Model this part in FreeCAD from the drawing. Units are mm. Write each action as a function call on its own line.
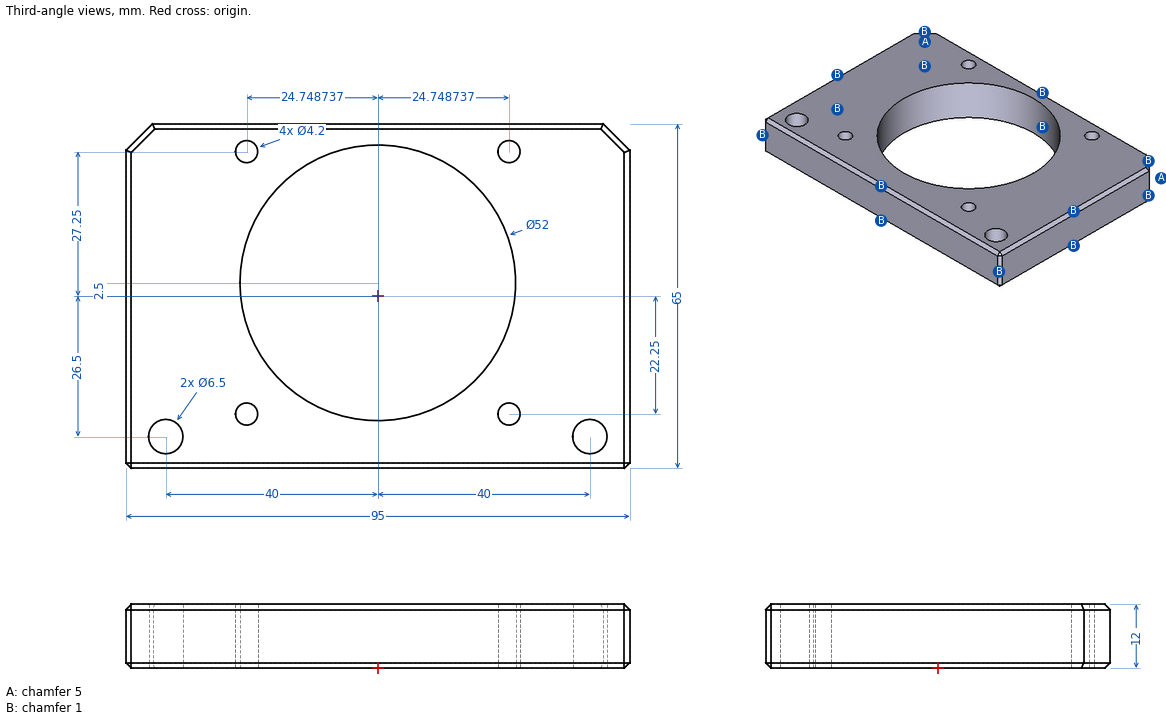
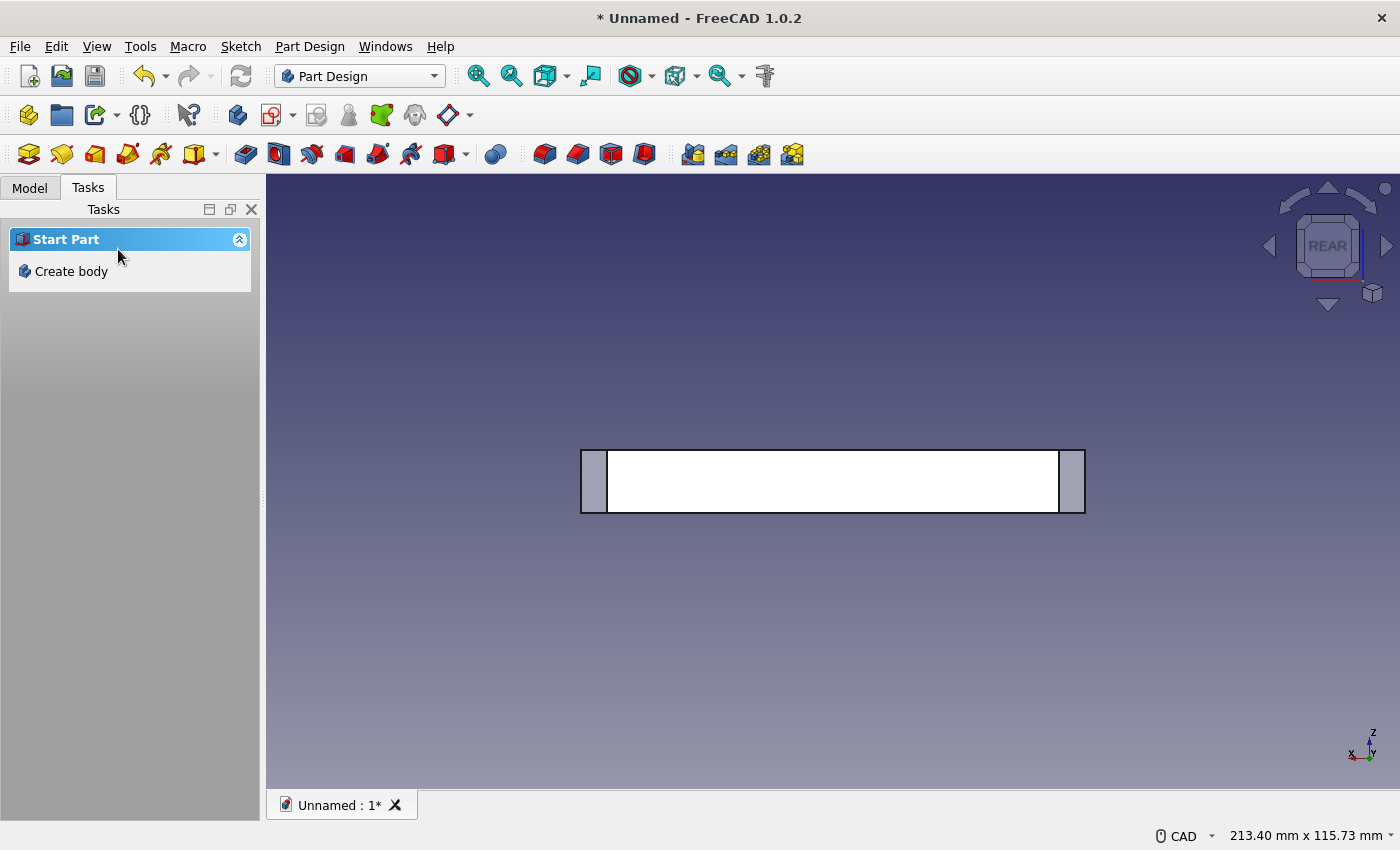
key(0)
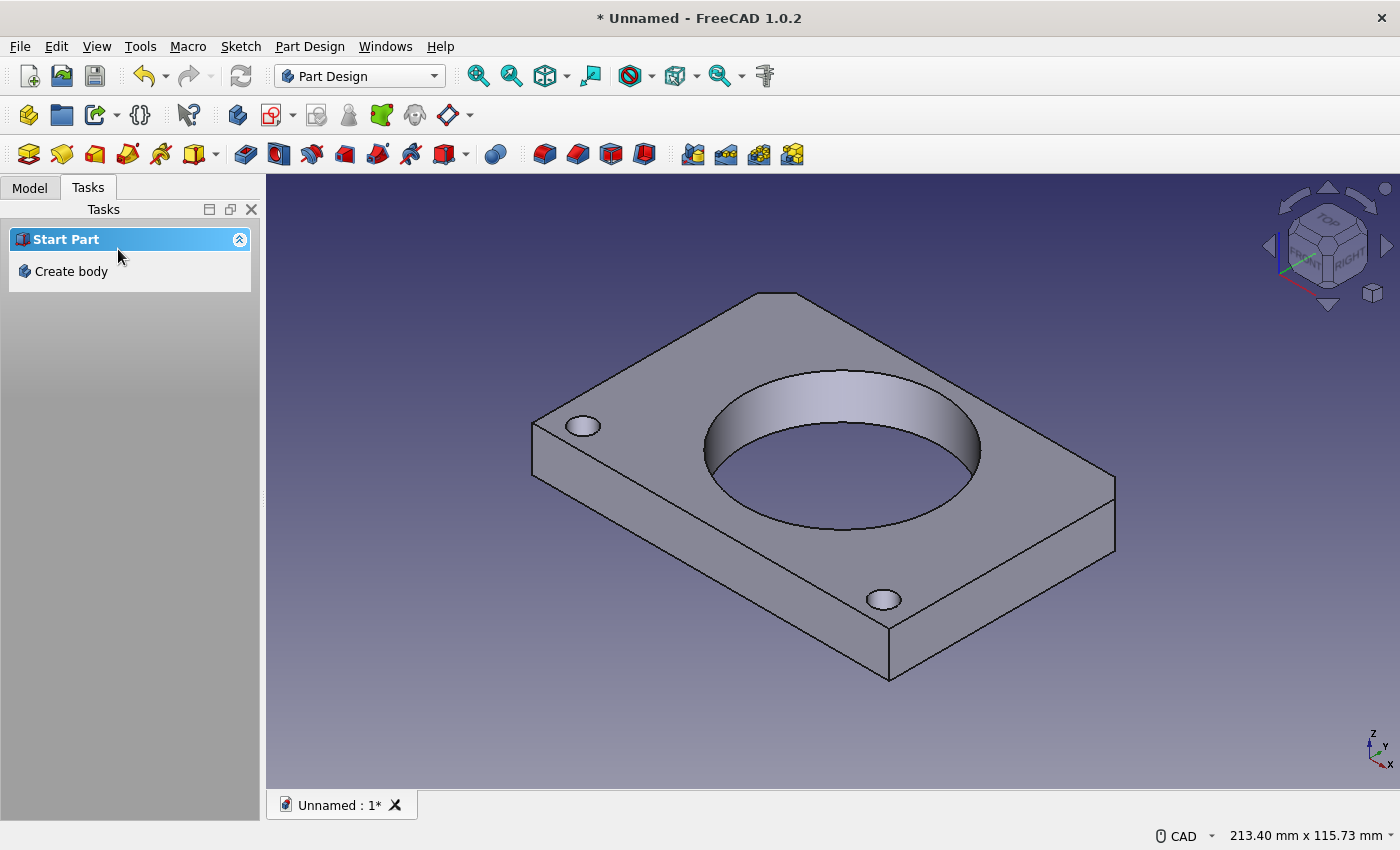
click(661, 436)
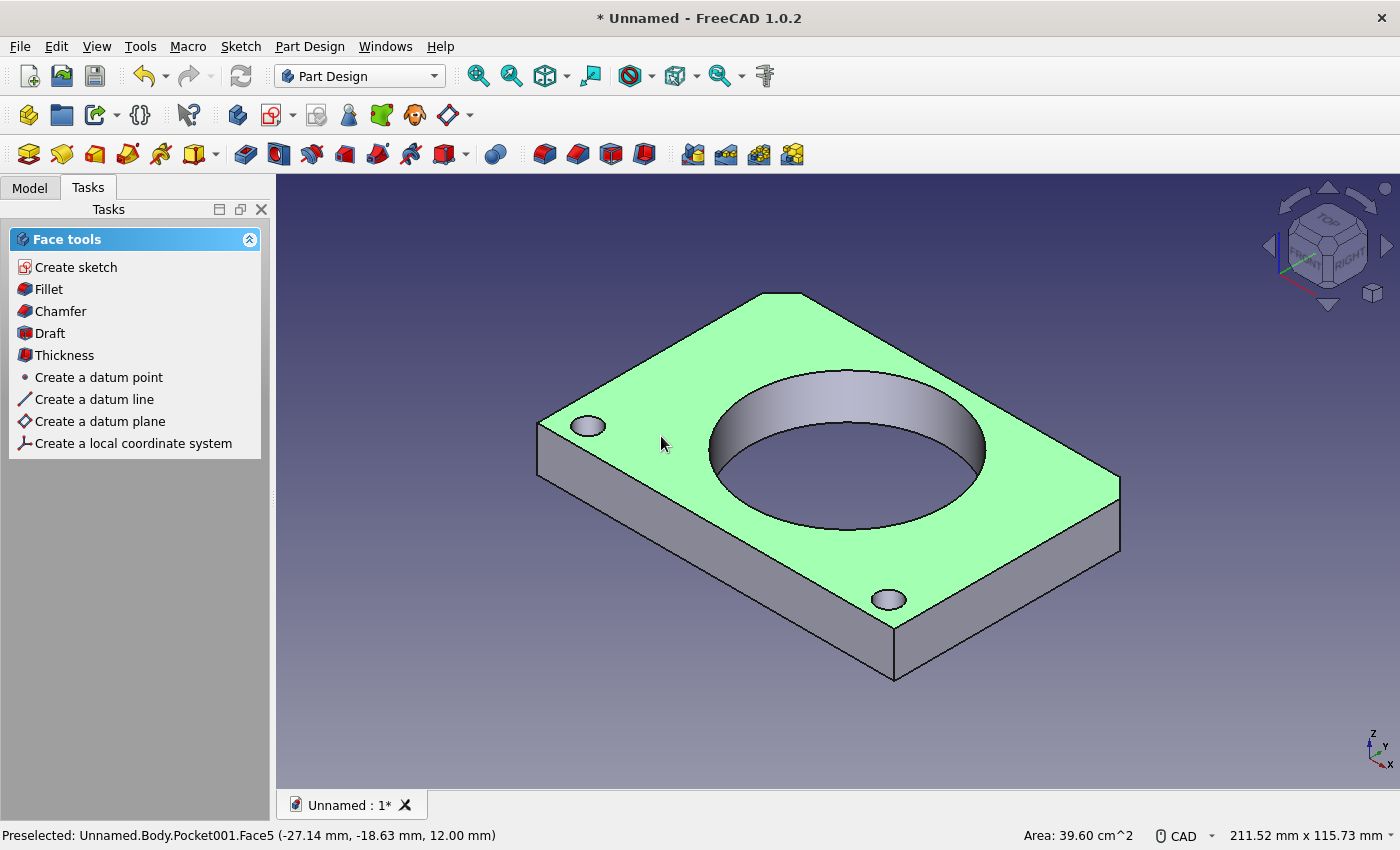
click(270, 116)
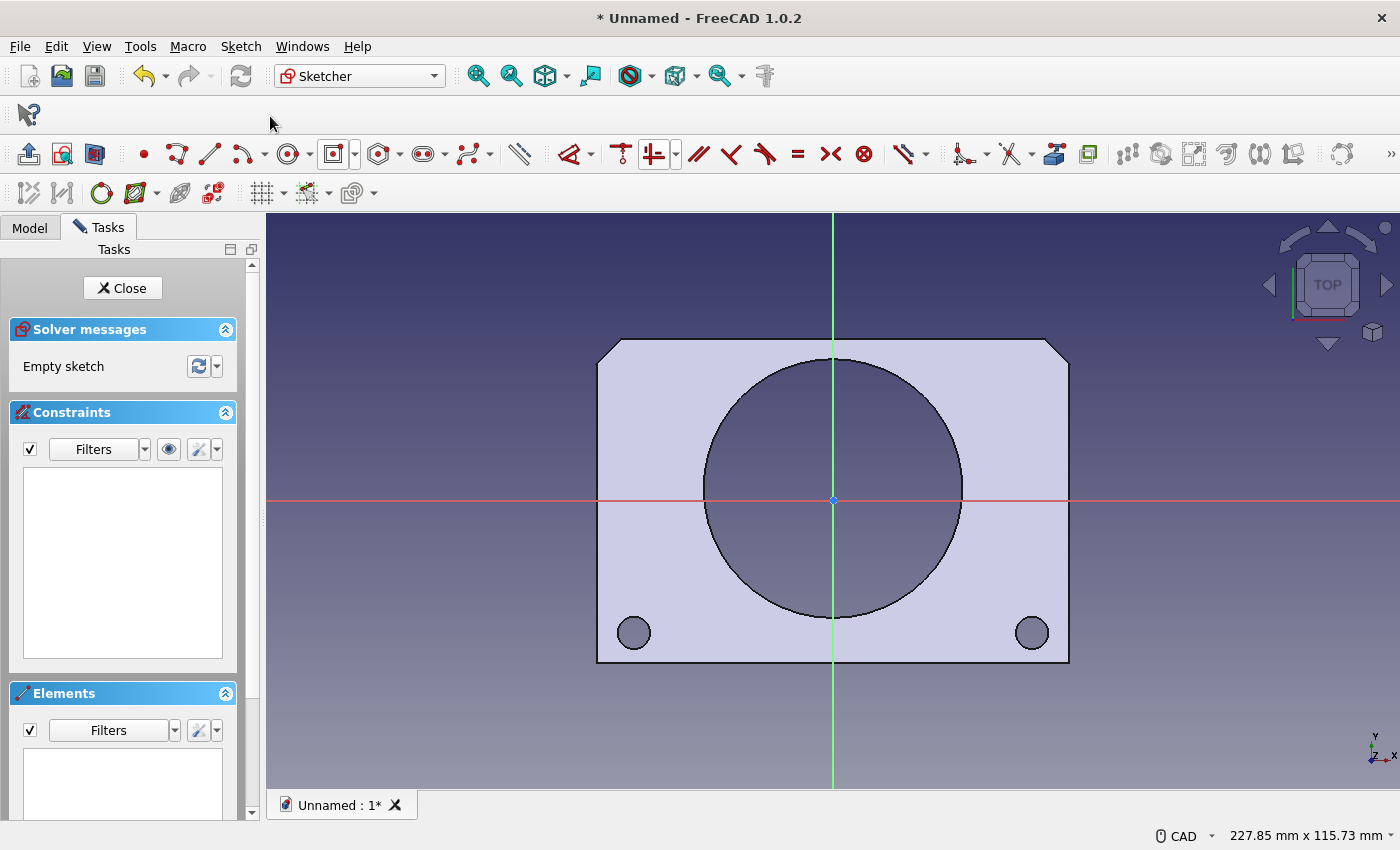
scroll(972, 463, up, 2)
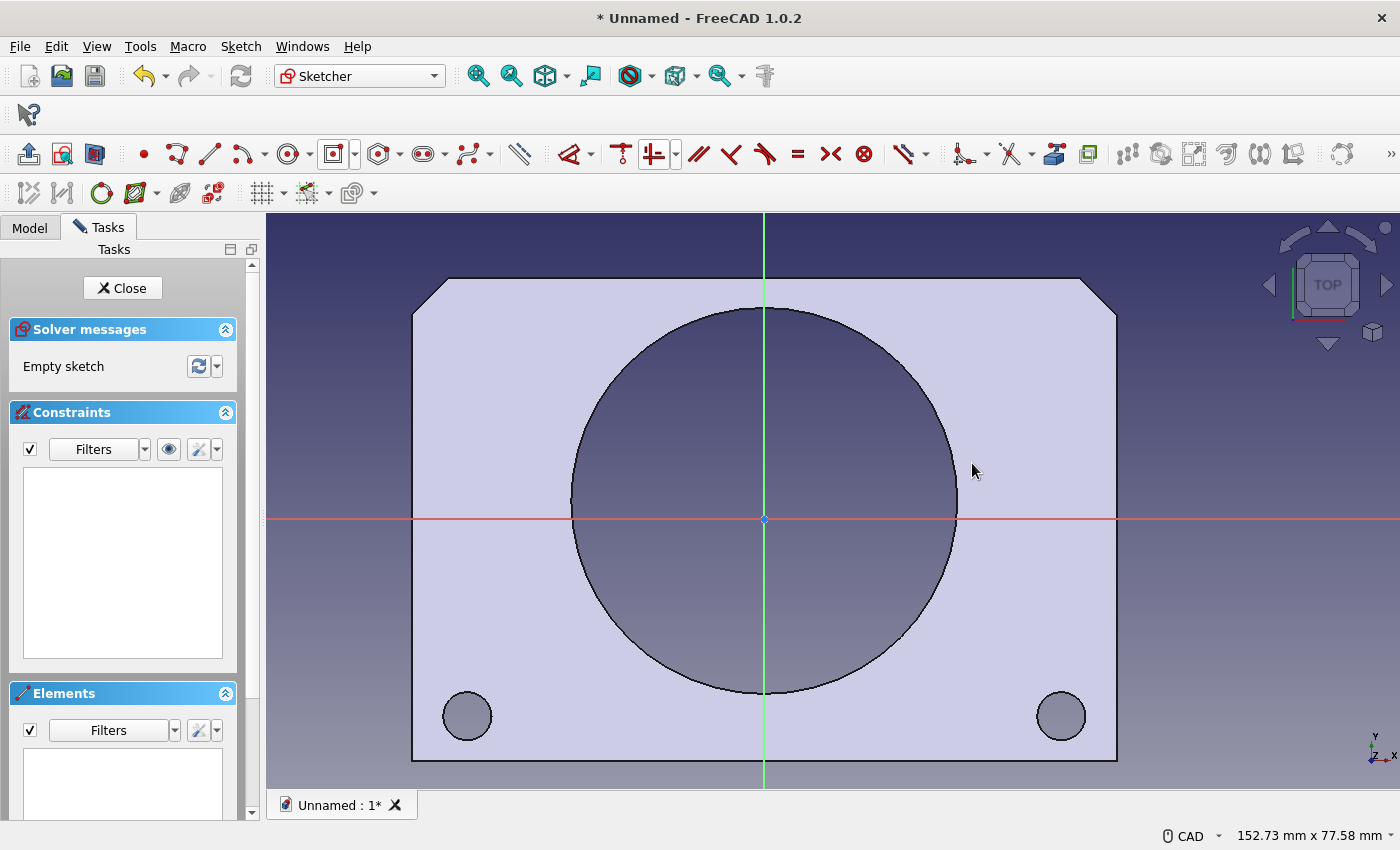
click(288, 154)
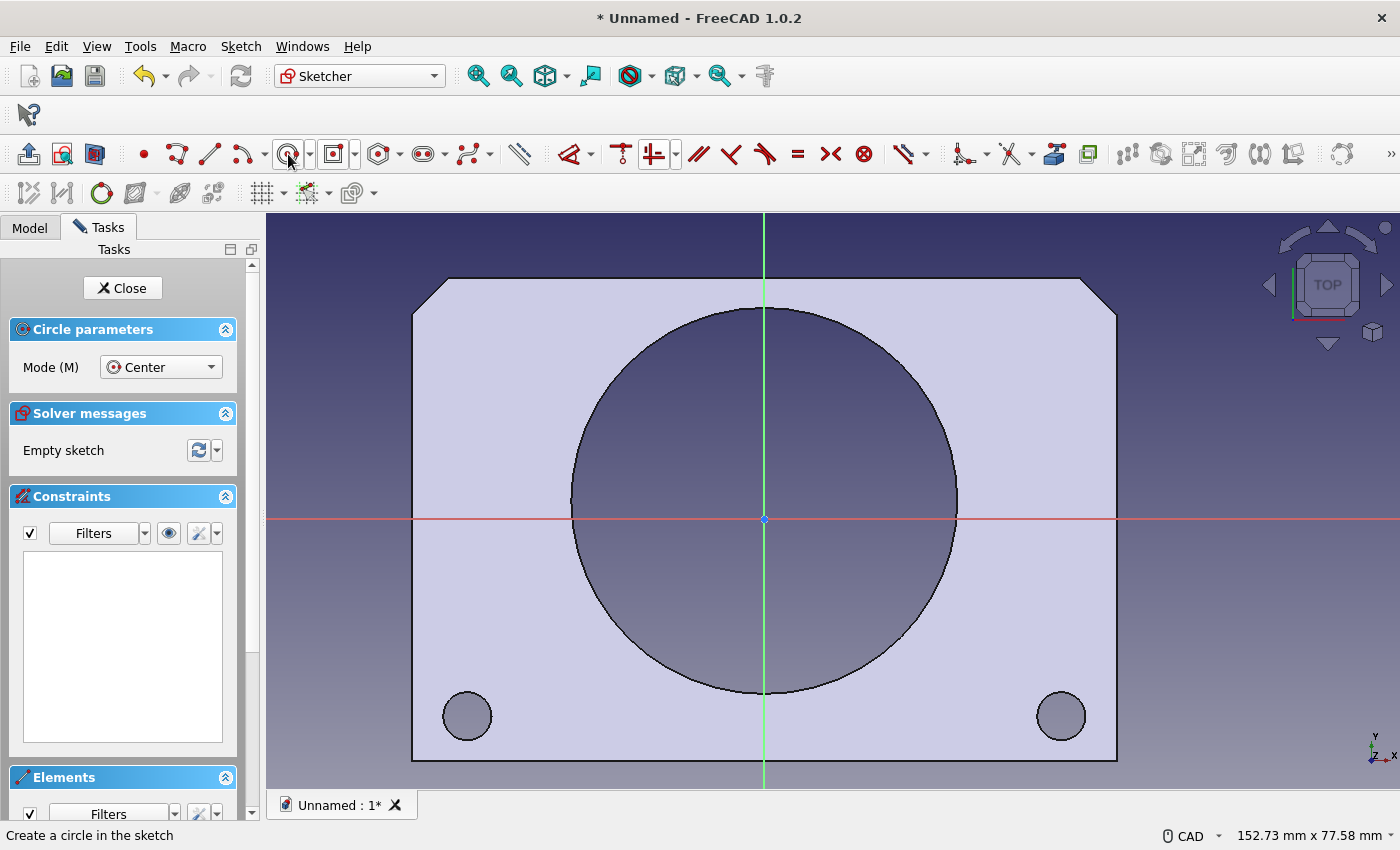
scroll(581, 317, up, 2)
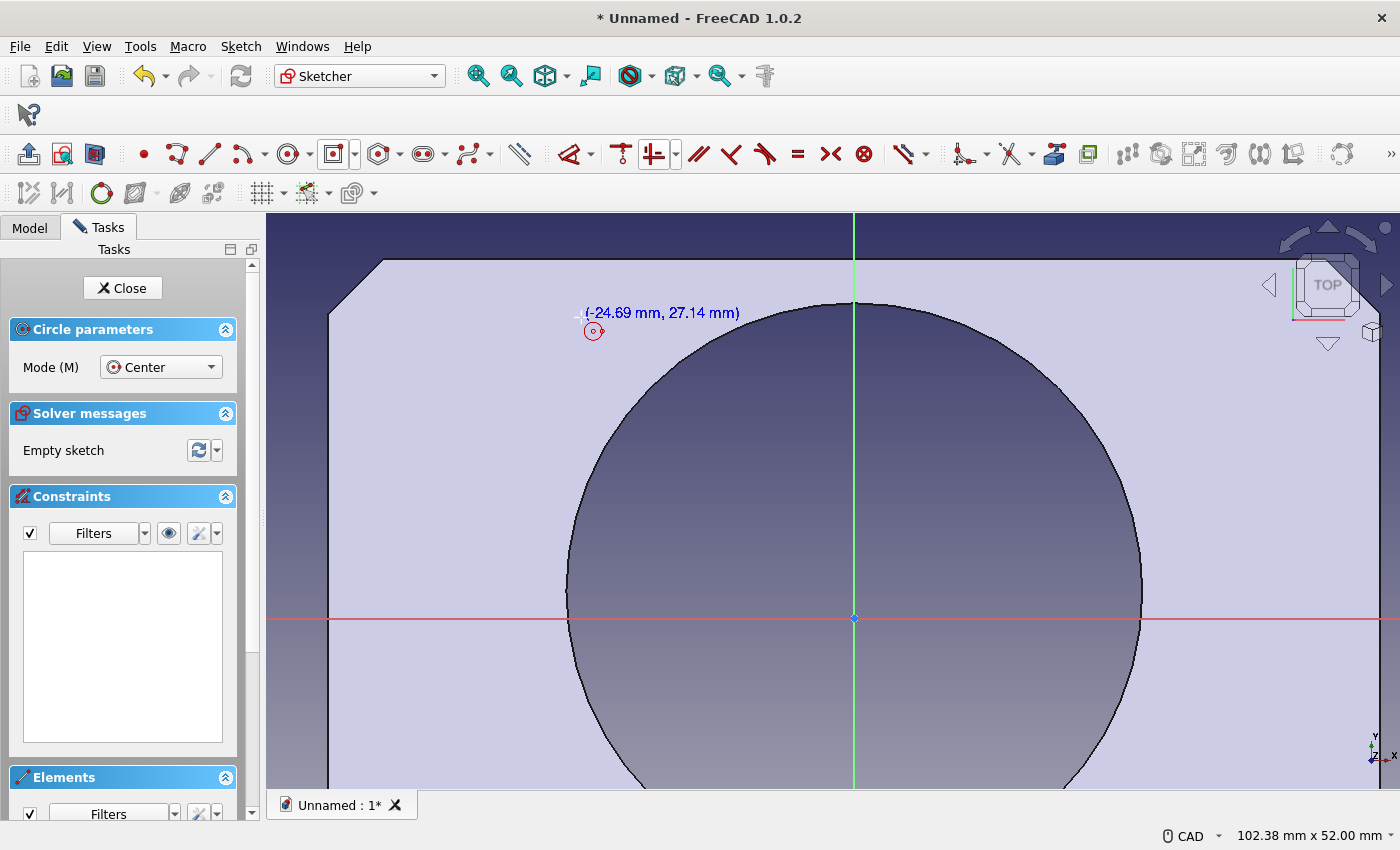
click(580, 317)
click(597, 301)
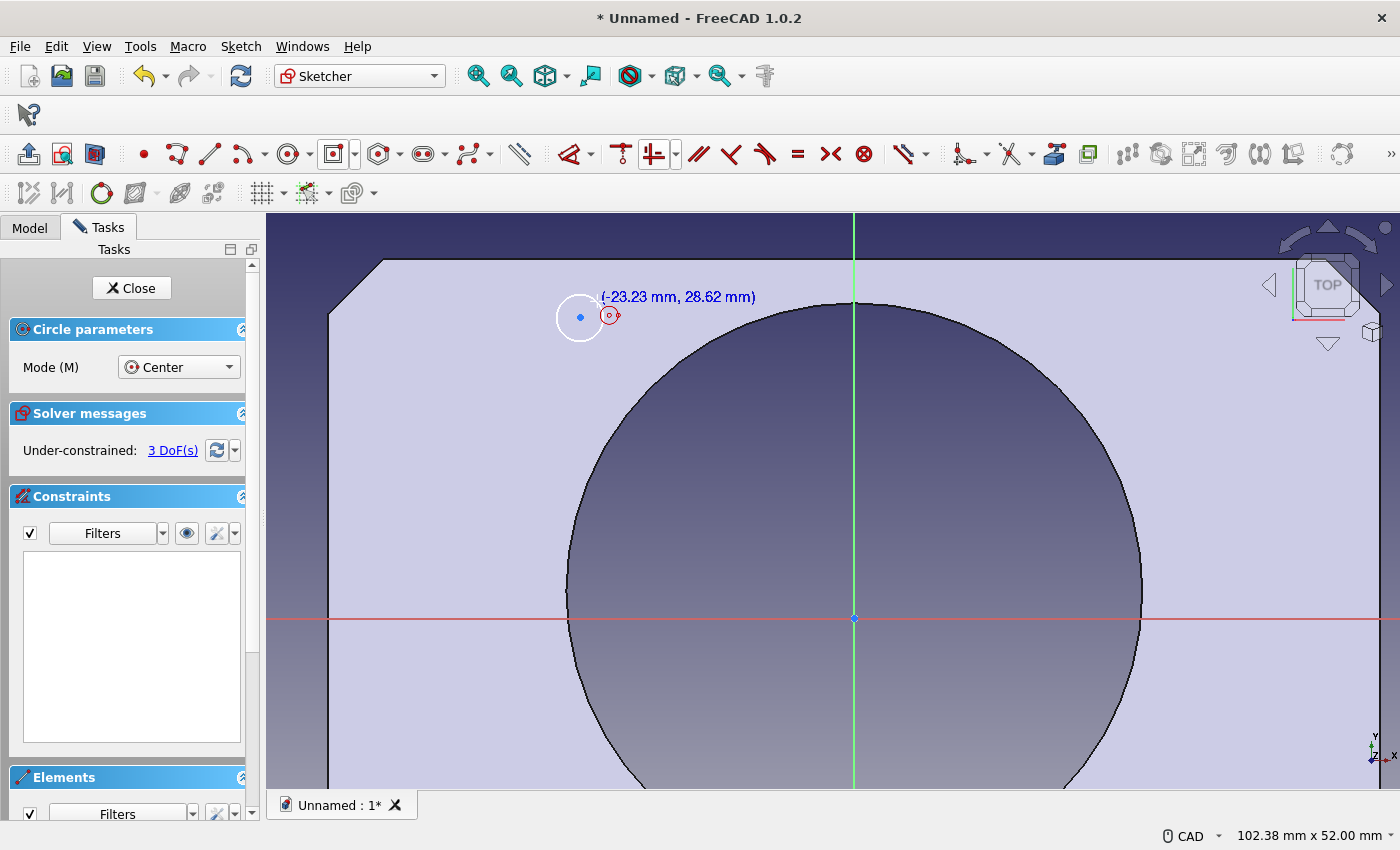
click(1128, 317)
click(1145, 301)